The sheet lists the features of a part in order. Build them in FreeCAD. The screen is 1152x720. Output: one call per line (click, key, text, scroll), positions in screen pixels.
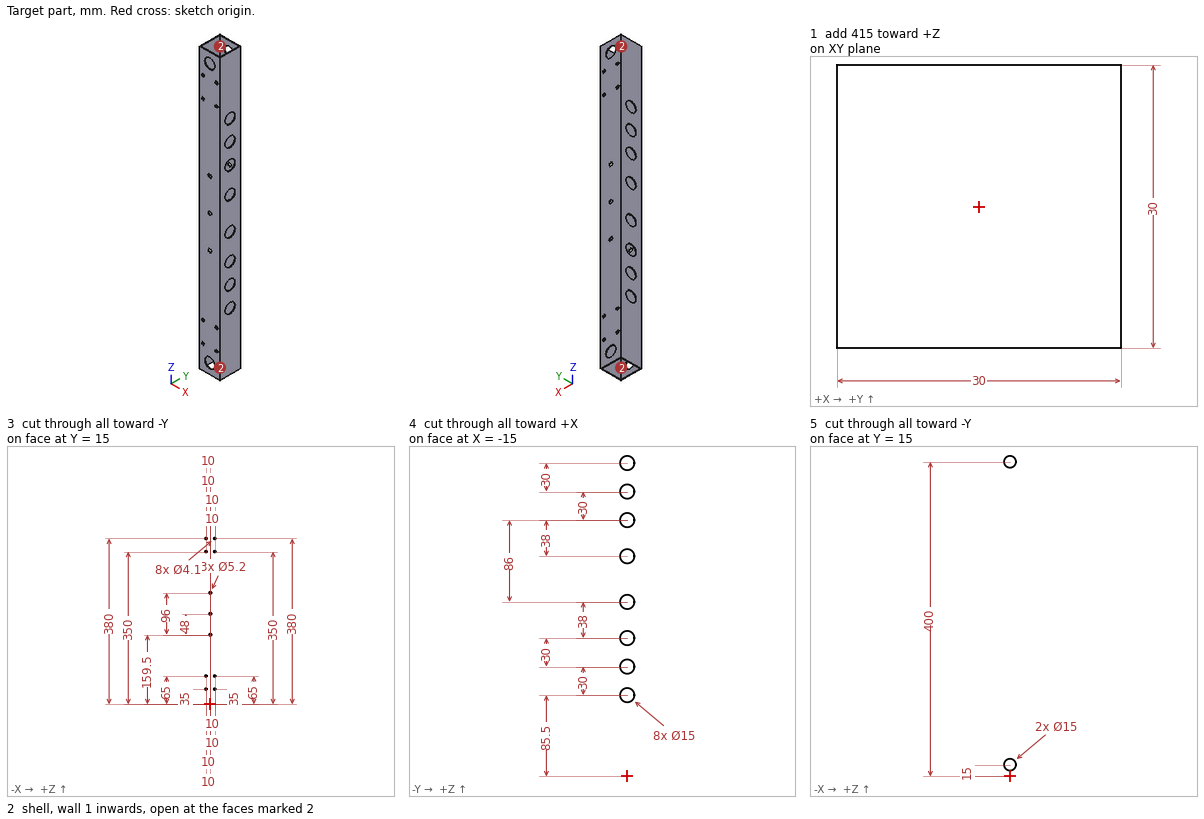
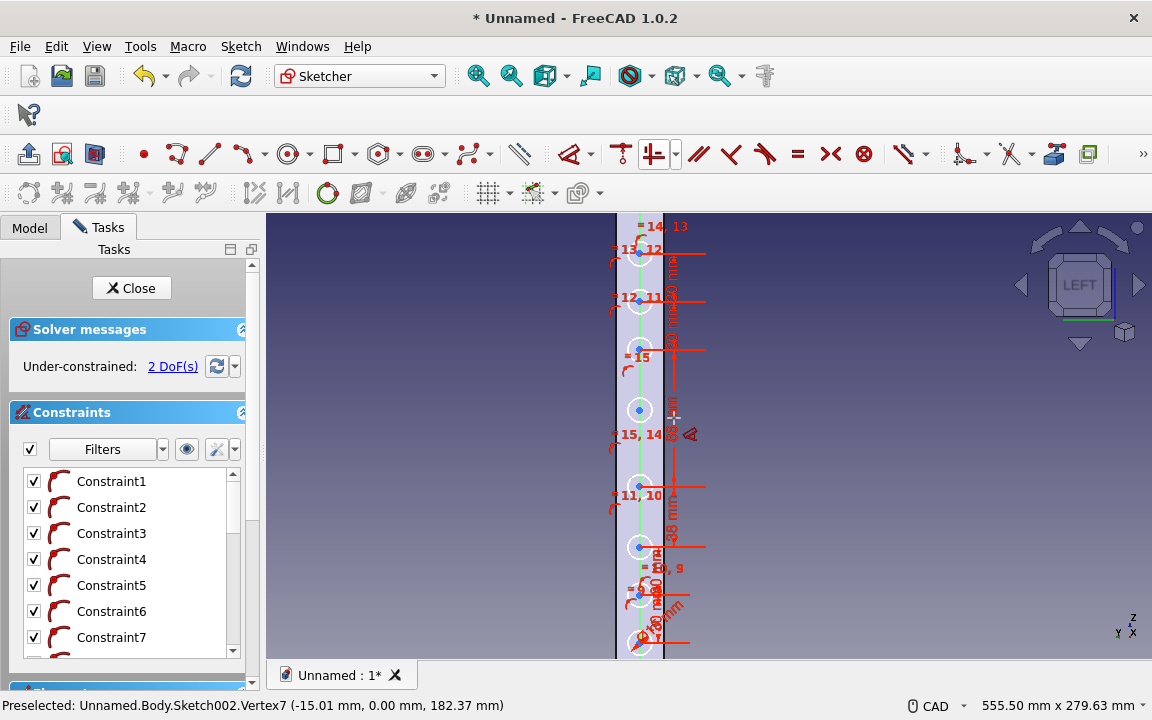
click(640, 350)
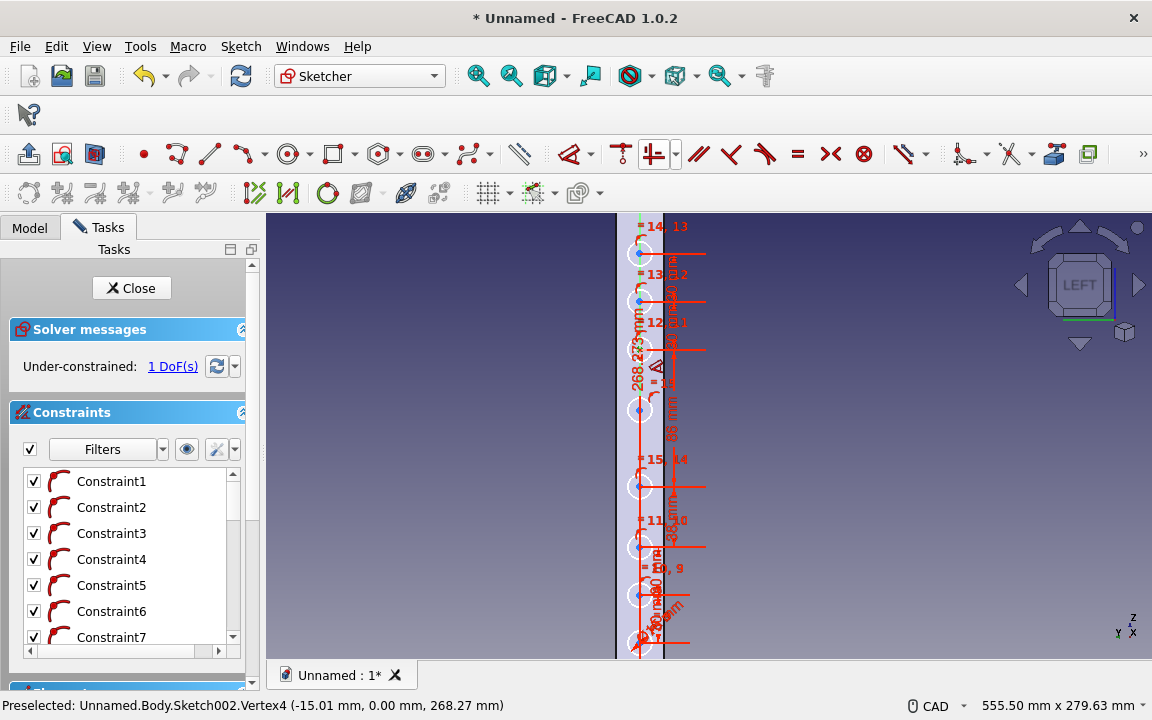
click(640, 410)
click(674, 380)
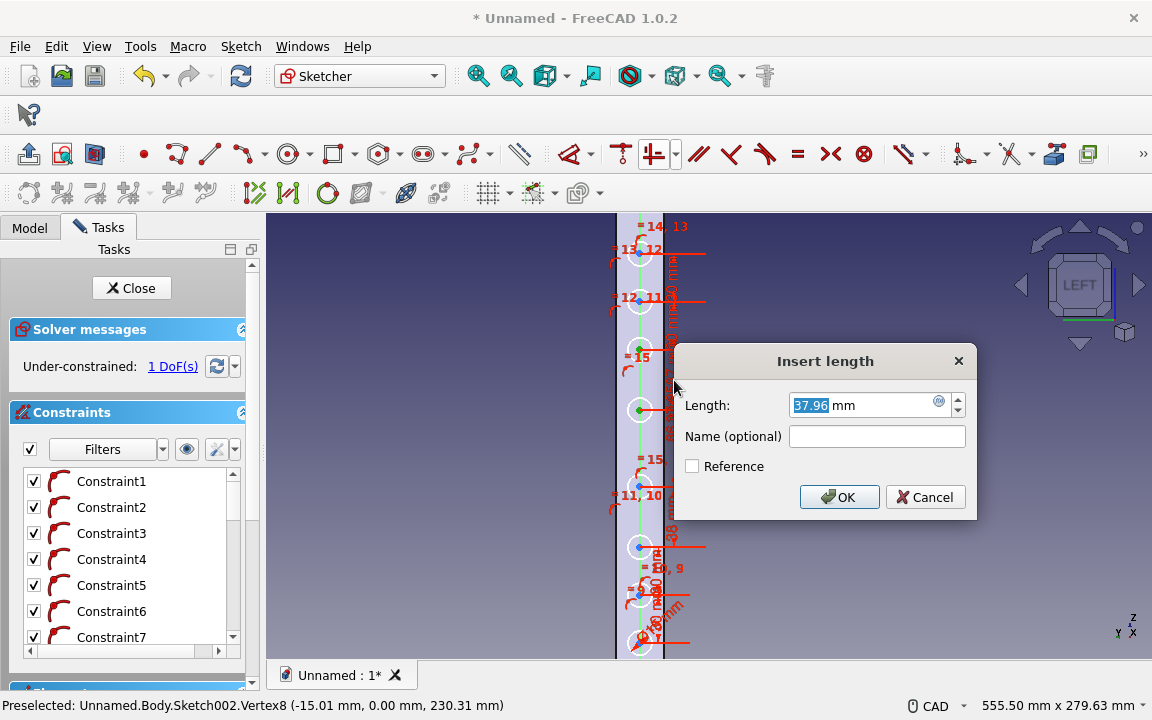
text(38)
key(Return)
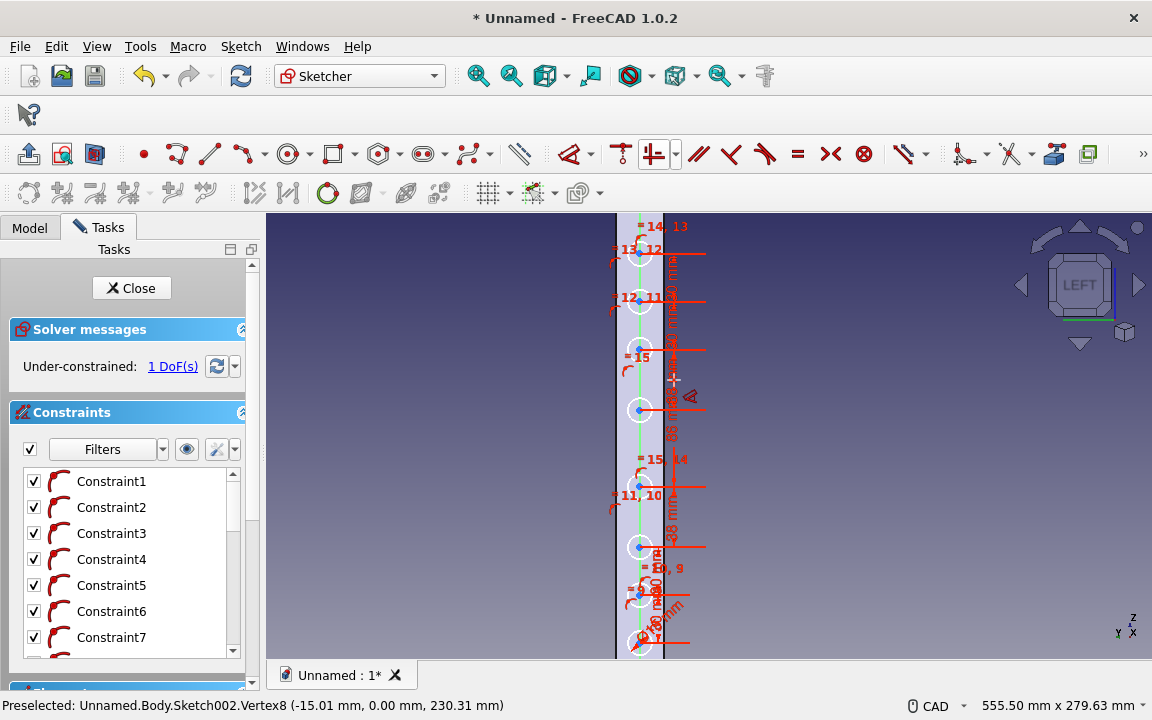
scroll(641, 348, down, 3)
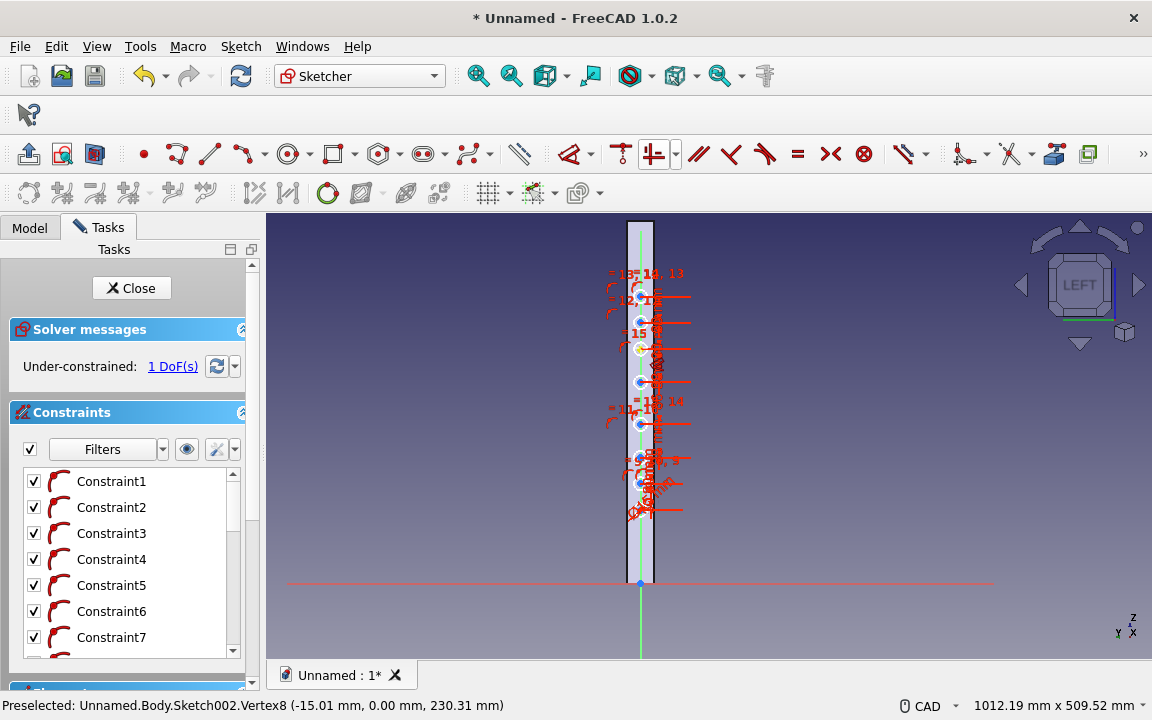
click(641, 510)
click(675, 547)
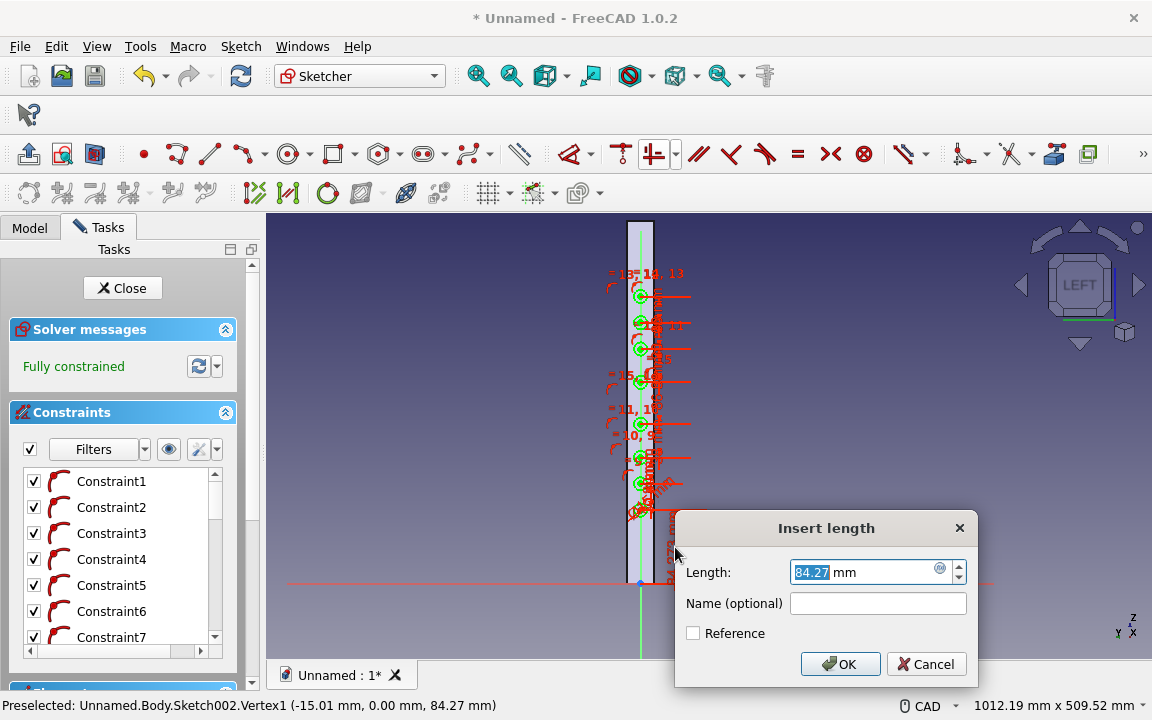
text(85.5)
key(Return)
key(Escape)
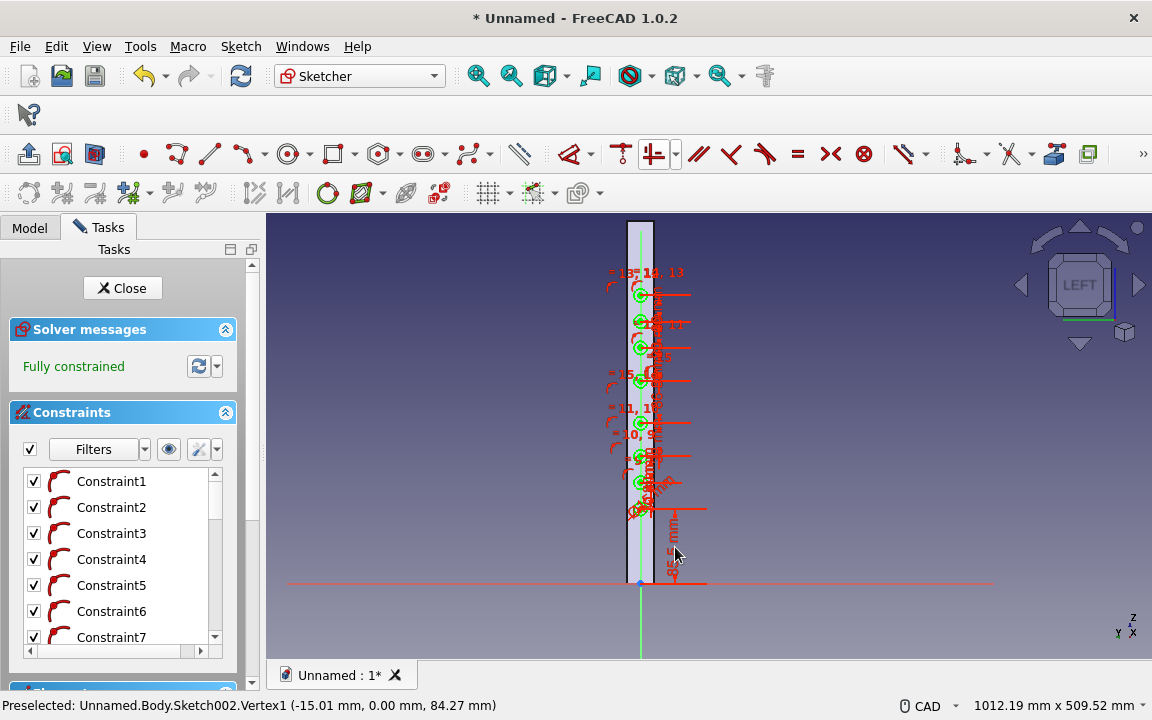
click(123, 288)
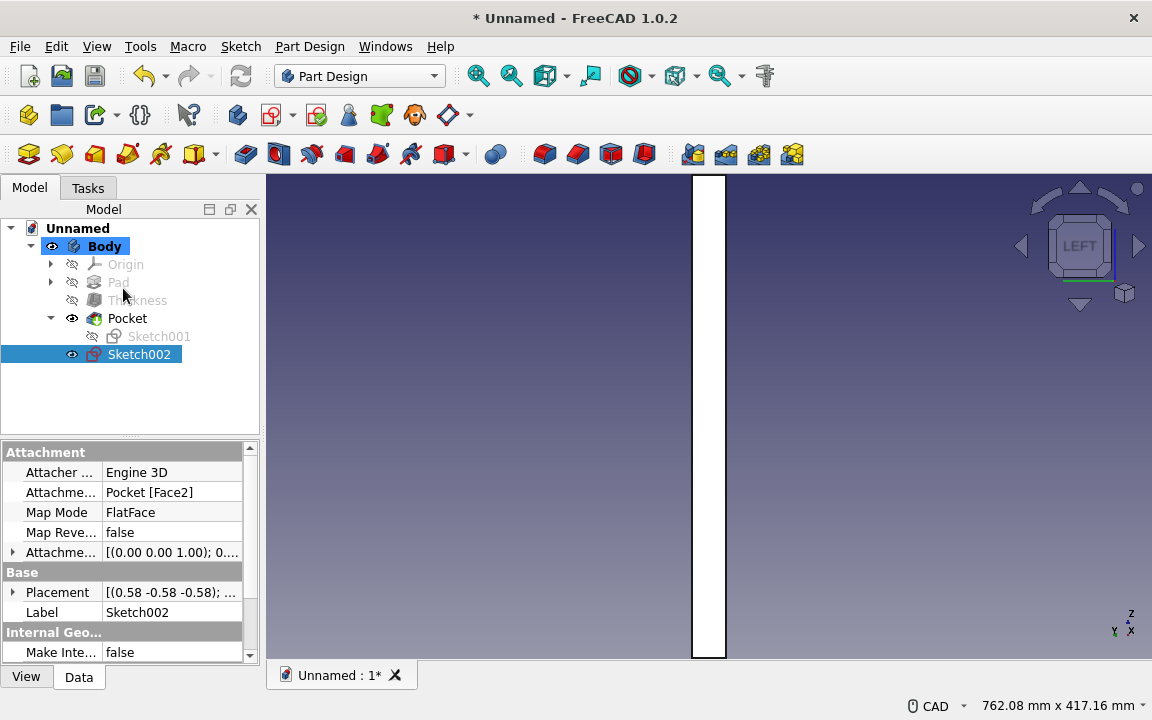
click(246, 154)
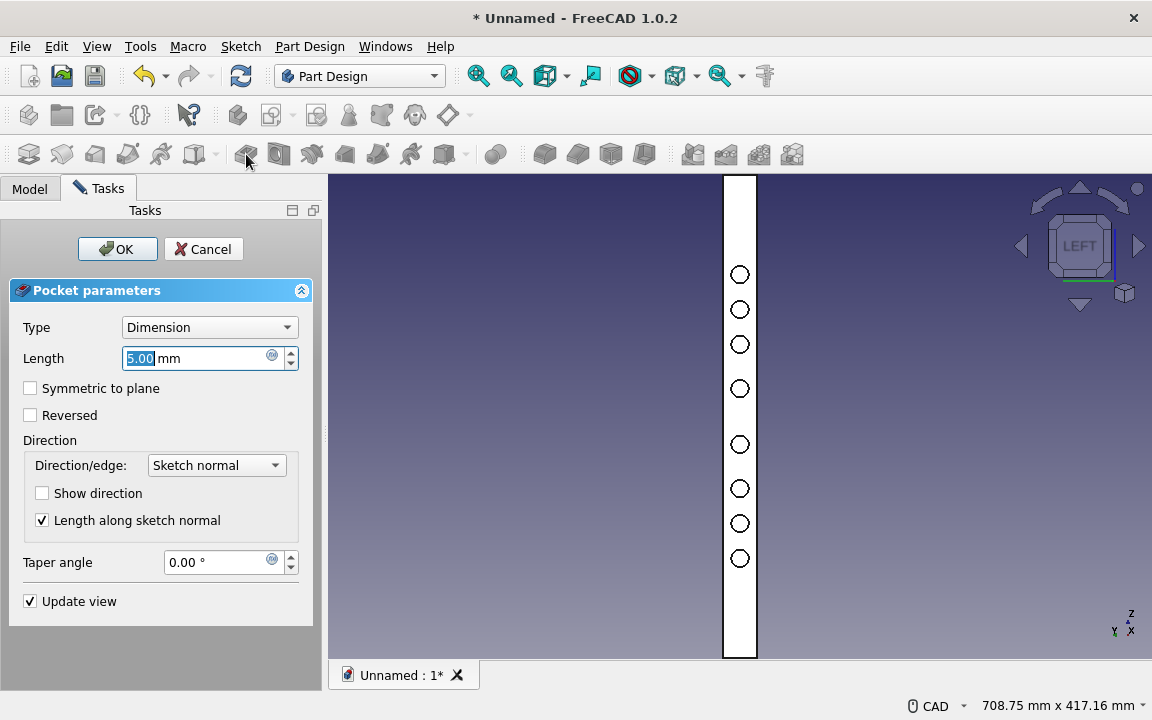
click(210, 328)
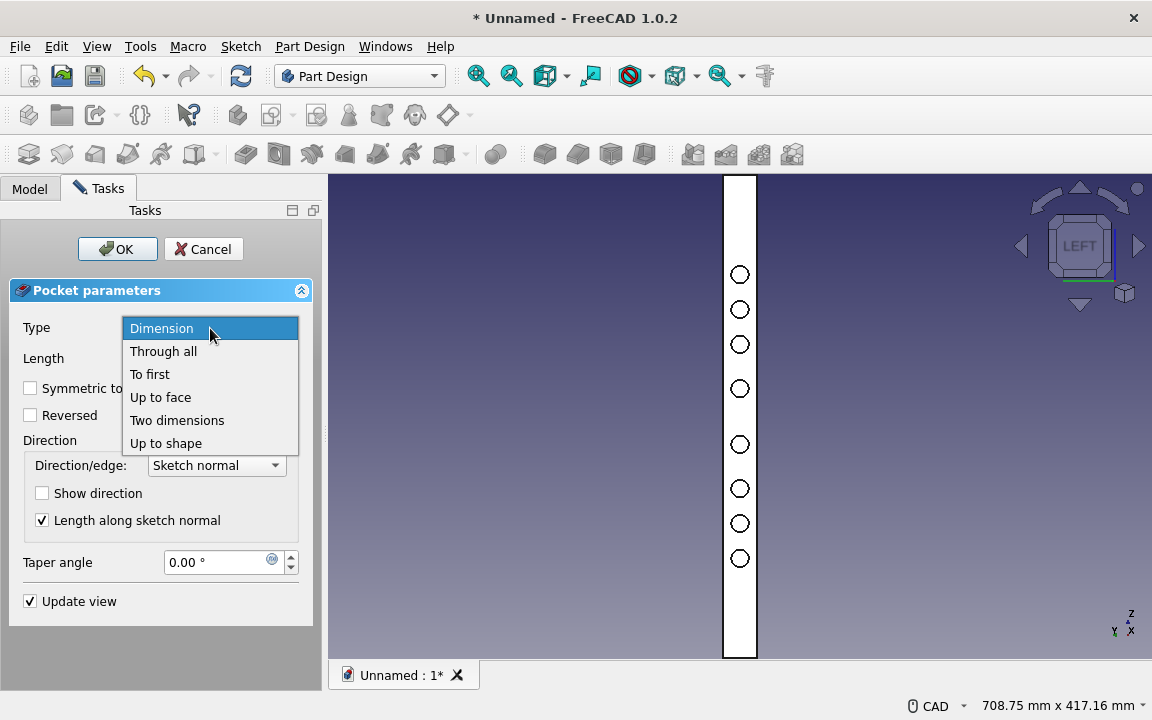
click(208, 352)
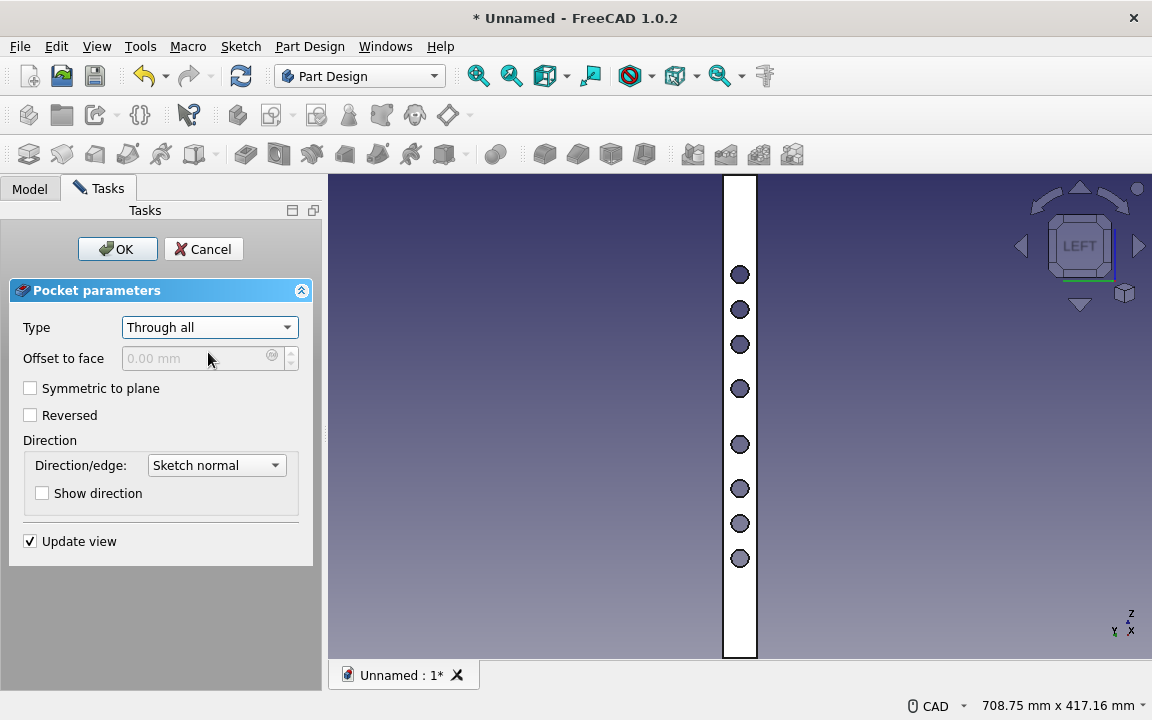
click(118, 249)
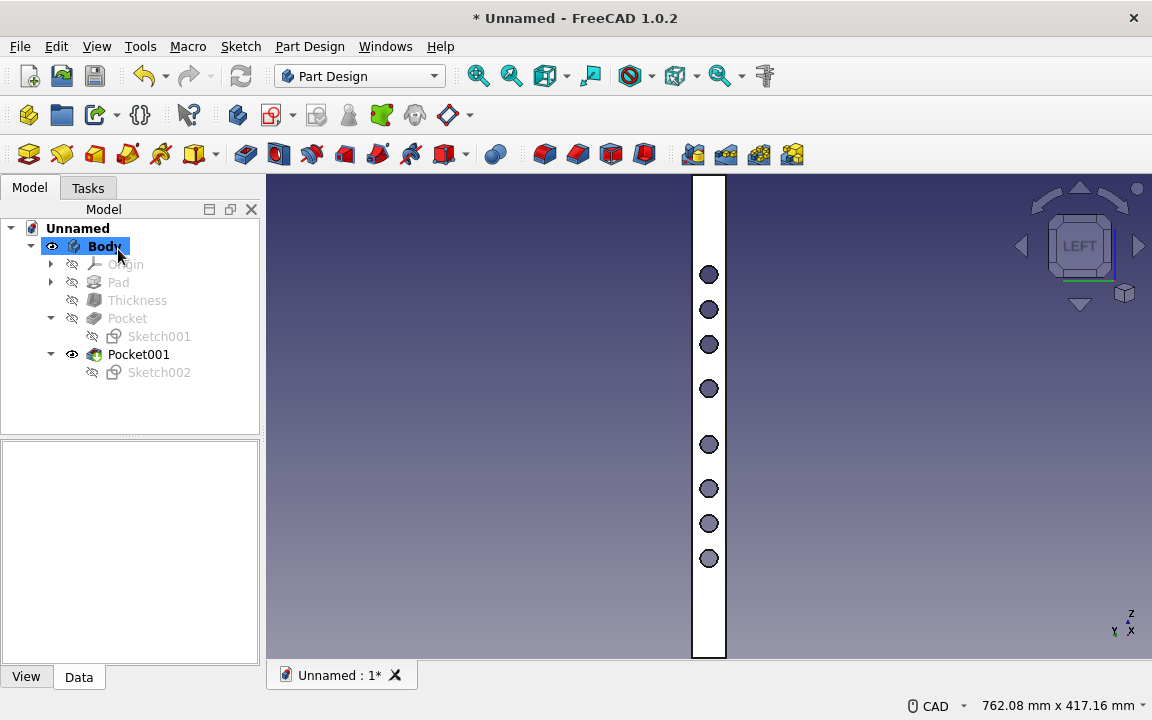
key(4)